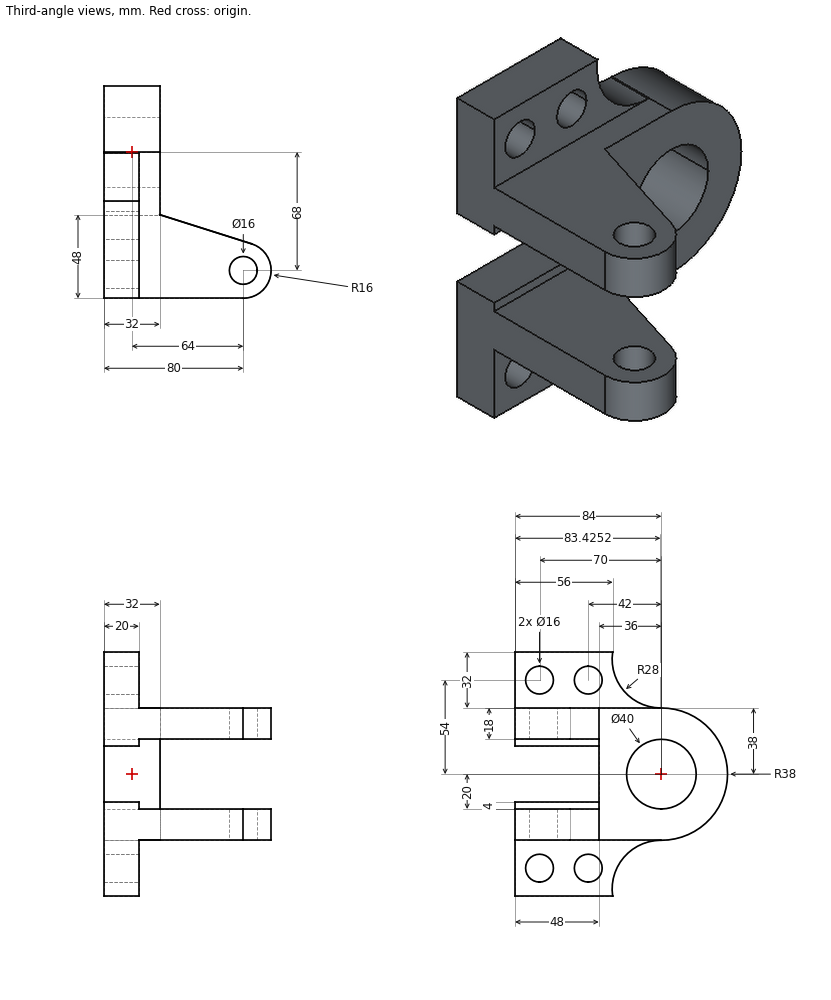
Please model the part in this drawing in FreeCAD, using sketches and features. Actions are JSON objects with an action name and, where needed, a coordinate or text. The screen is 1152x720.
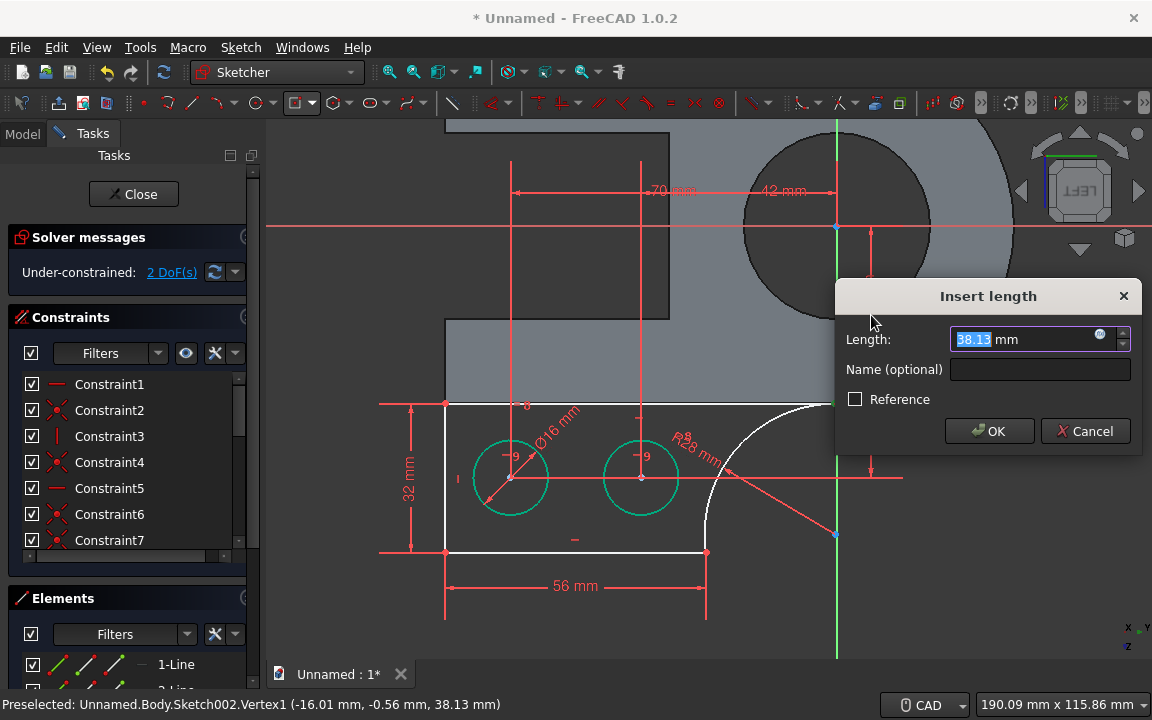
{"action": "type", "text": "38"}
{"action": "key", "text": "Return"}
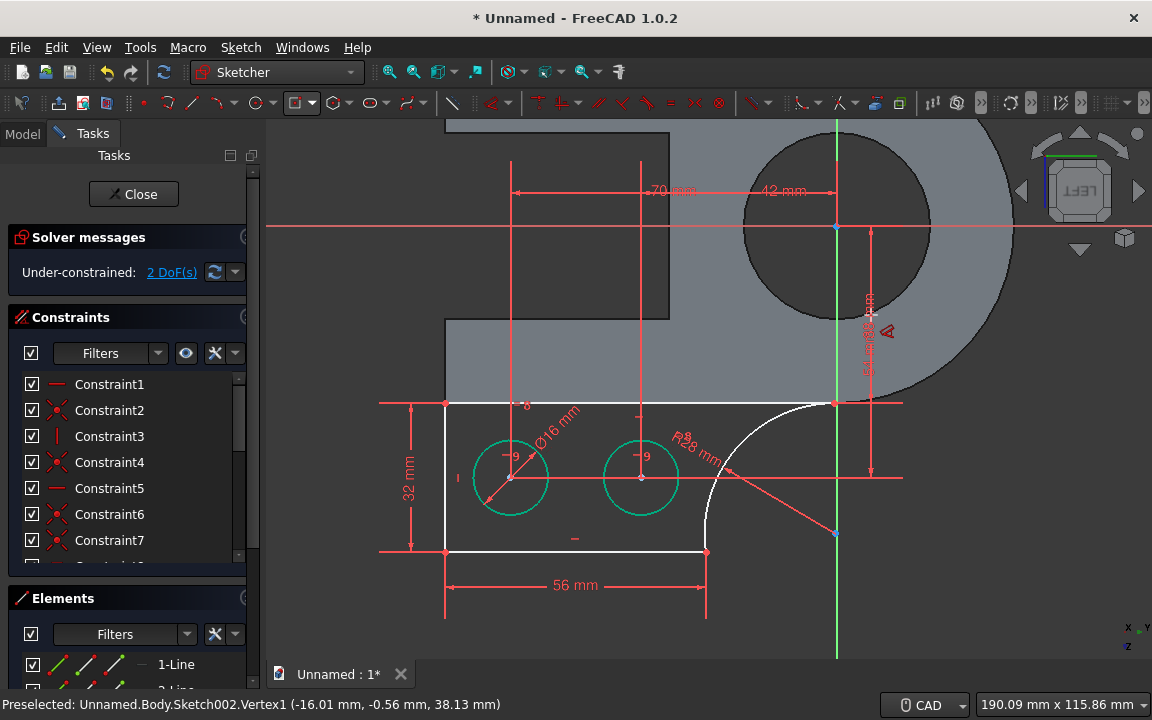
{"action": "left_click", "coordinate": [445, 403]}
{"action": "left_click", "coordinate": [551, 192]}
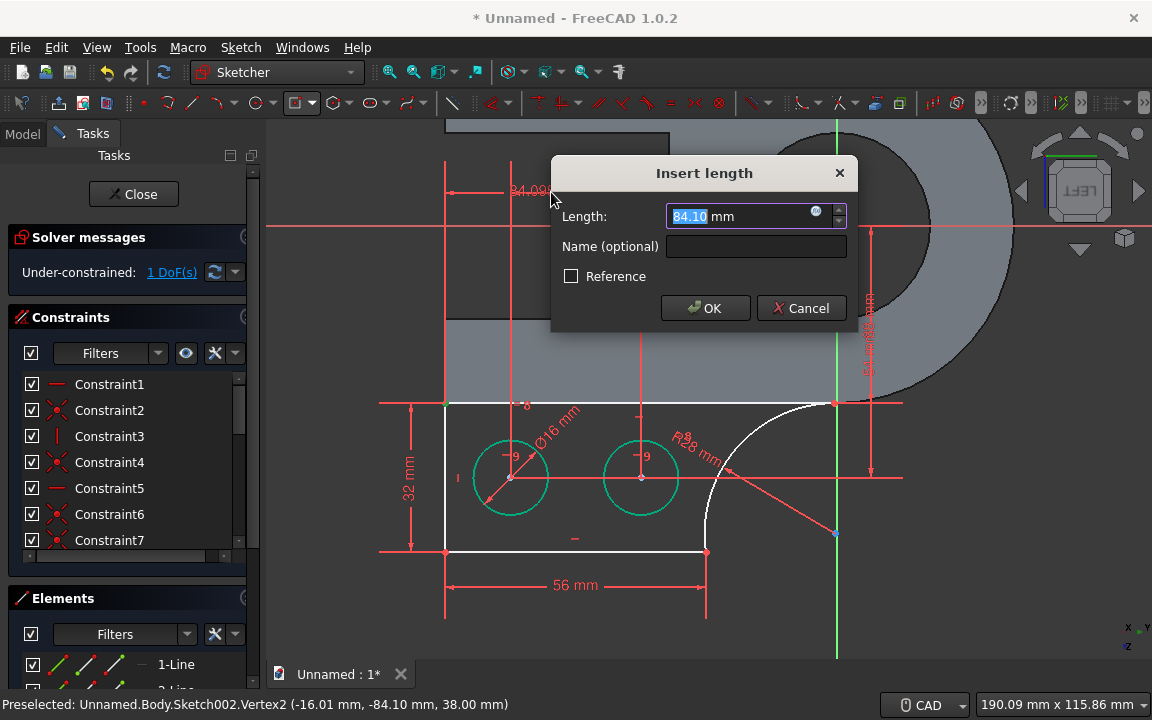
{"action": "type", "text": "84"}
{"action": "key", "text": "Return"}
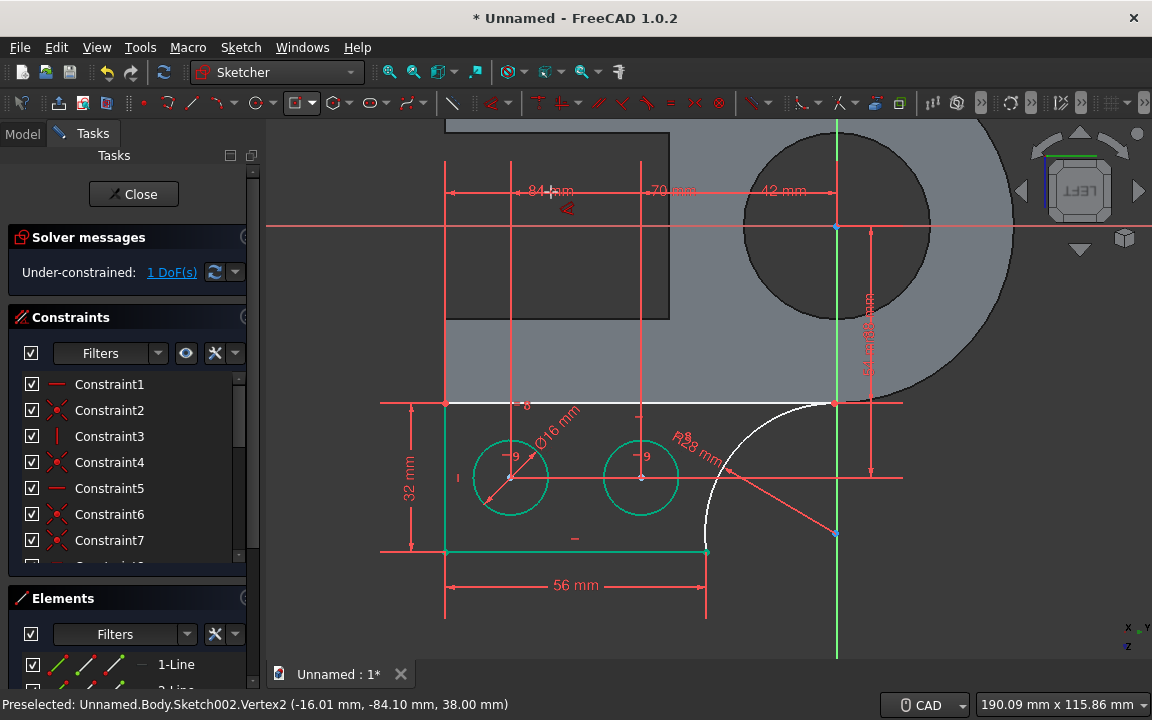
{"action": "left_click", "coordinate": [718, 403]}
{"action": "left_click", "coordinate": [776, 437]}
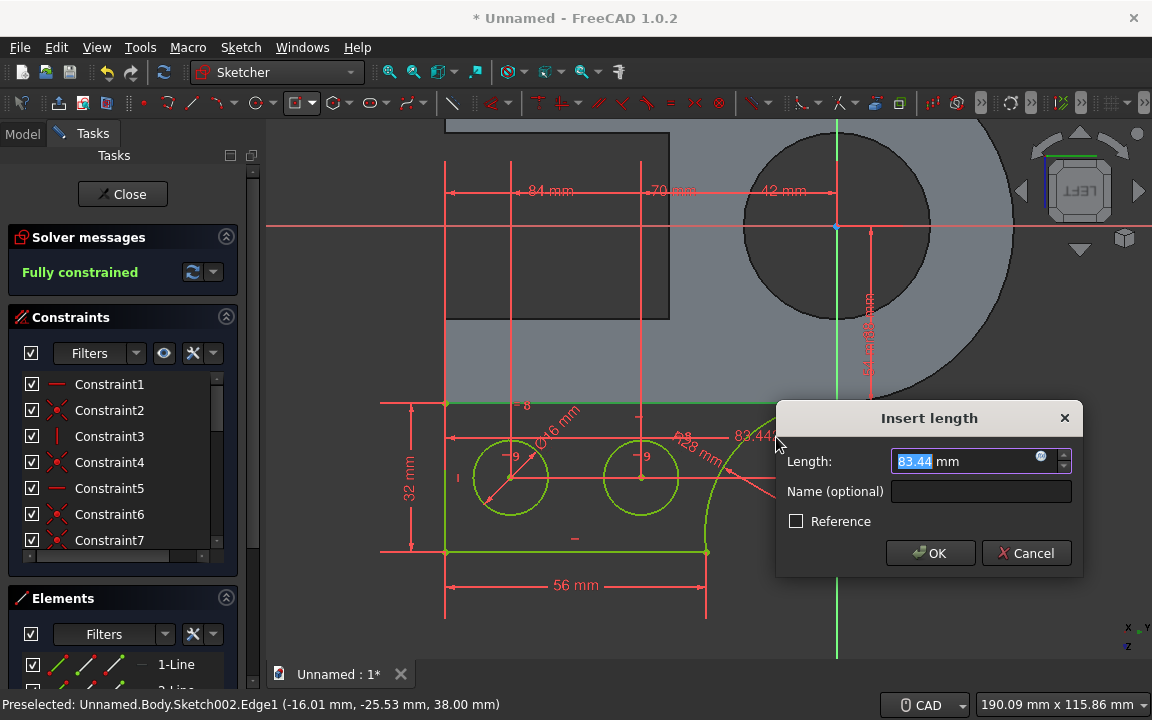
{"action": "type", "text": "83.4252"}
{"action": "key", "text": "Return"}
{"action": "key", "text": "Escape"}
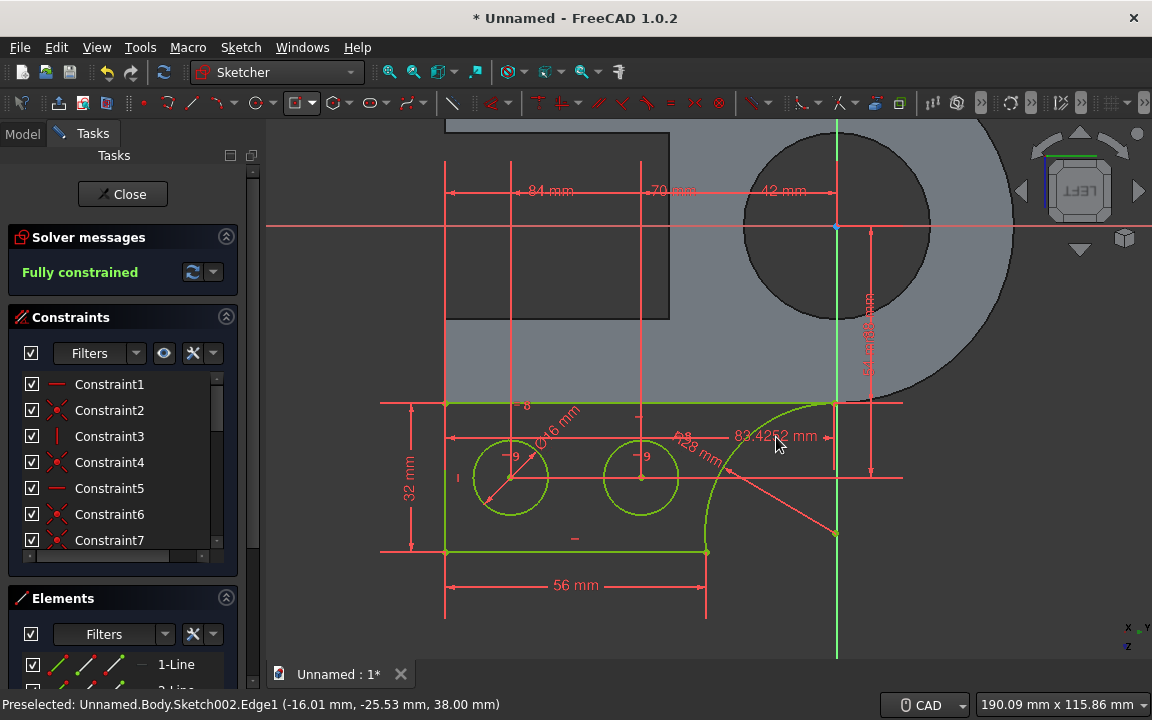
{"action": "left_click", "coordinate": [123, 194]}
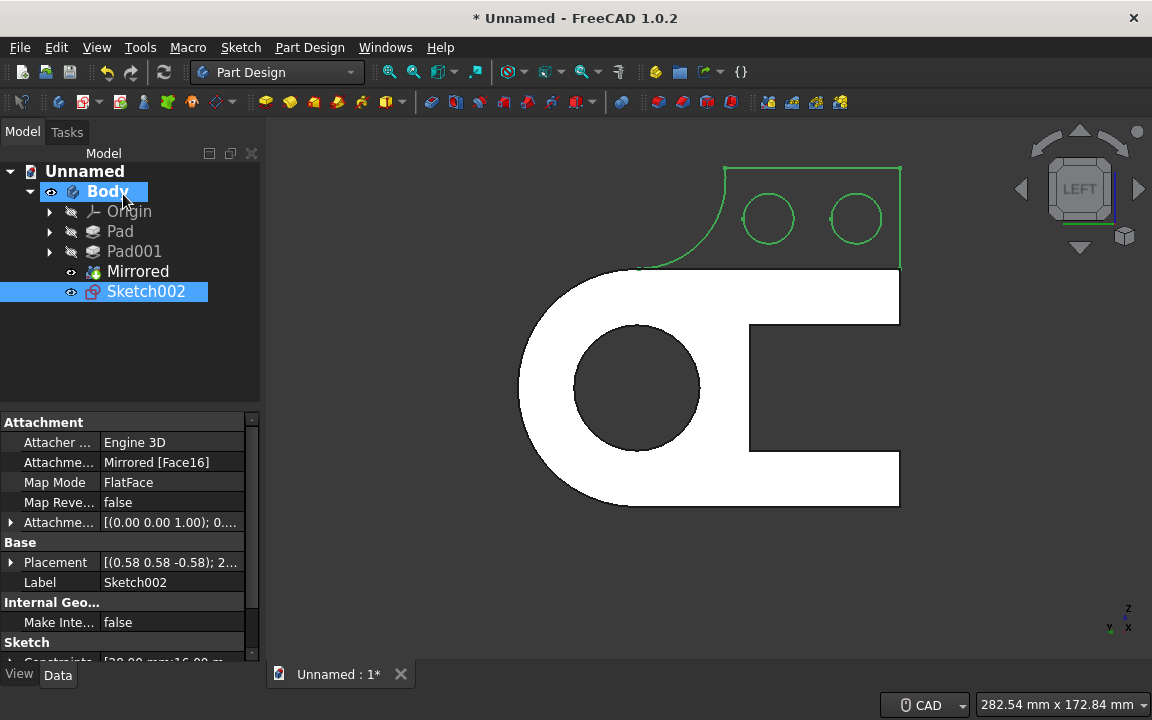
{"action": "left_click", "coordinate": [266, 102]}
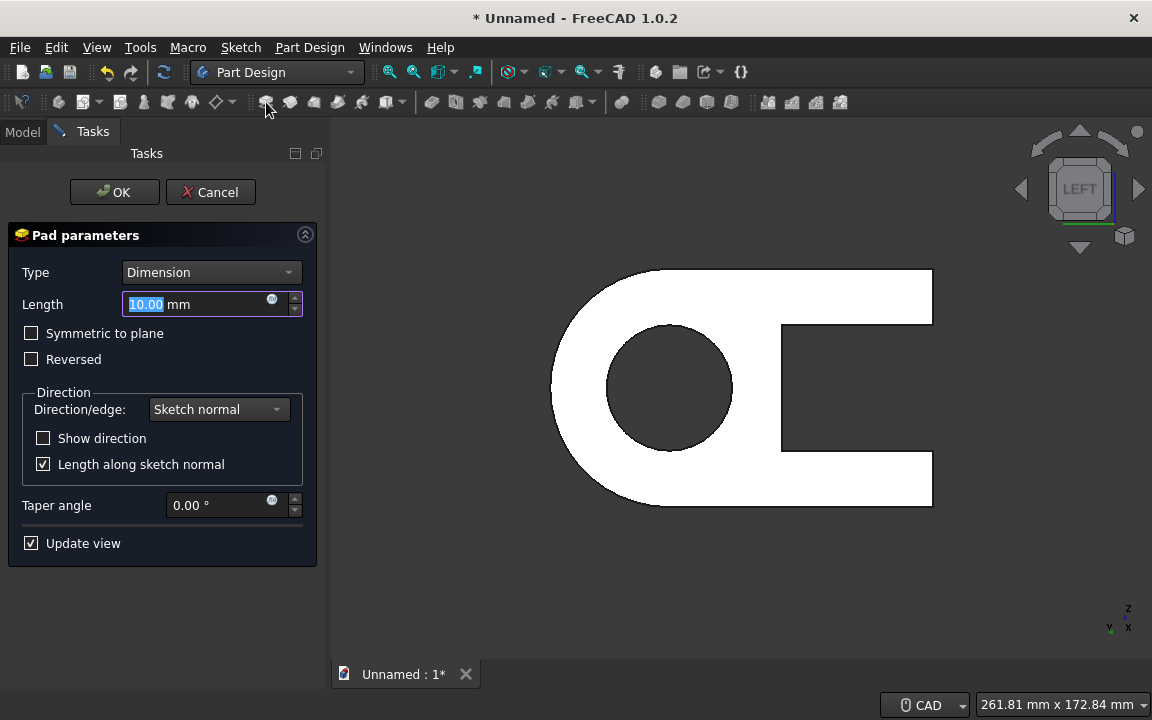
{"action": "type", "text": "20"}
{"action": "key", "text": "Tab"}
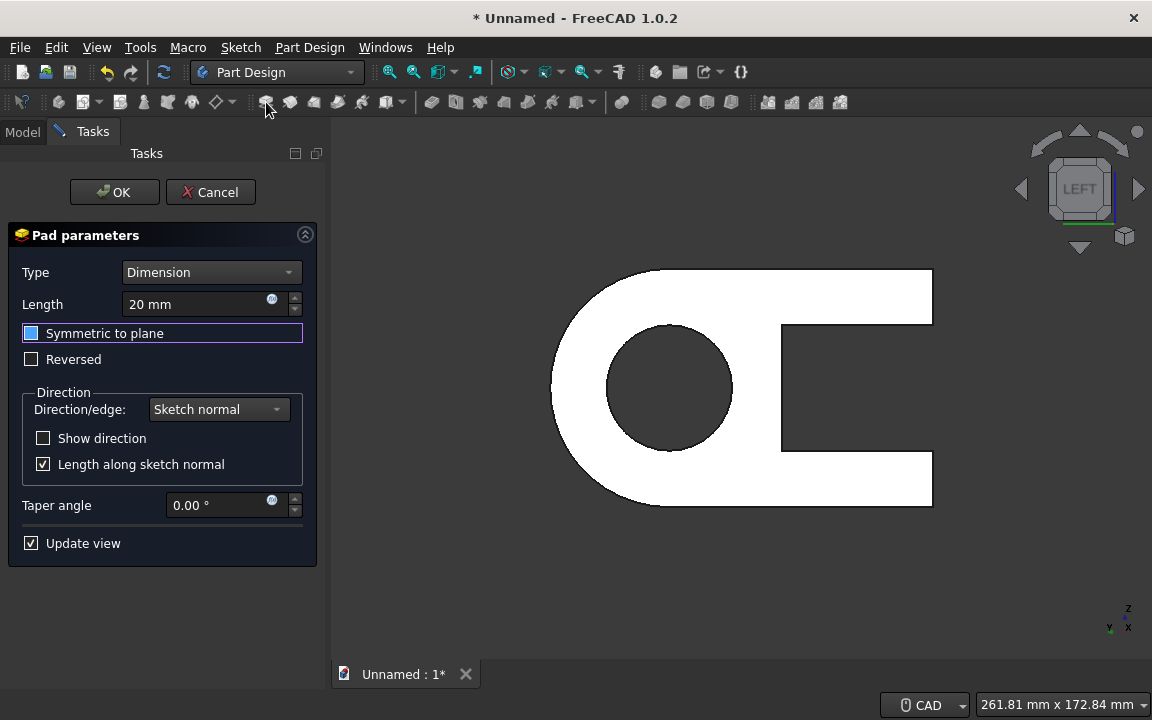
{"action": "left_click", "coordinate": [30, 359]}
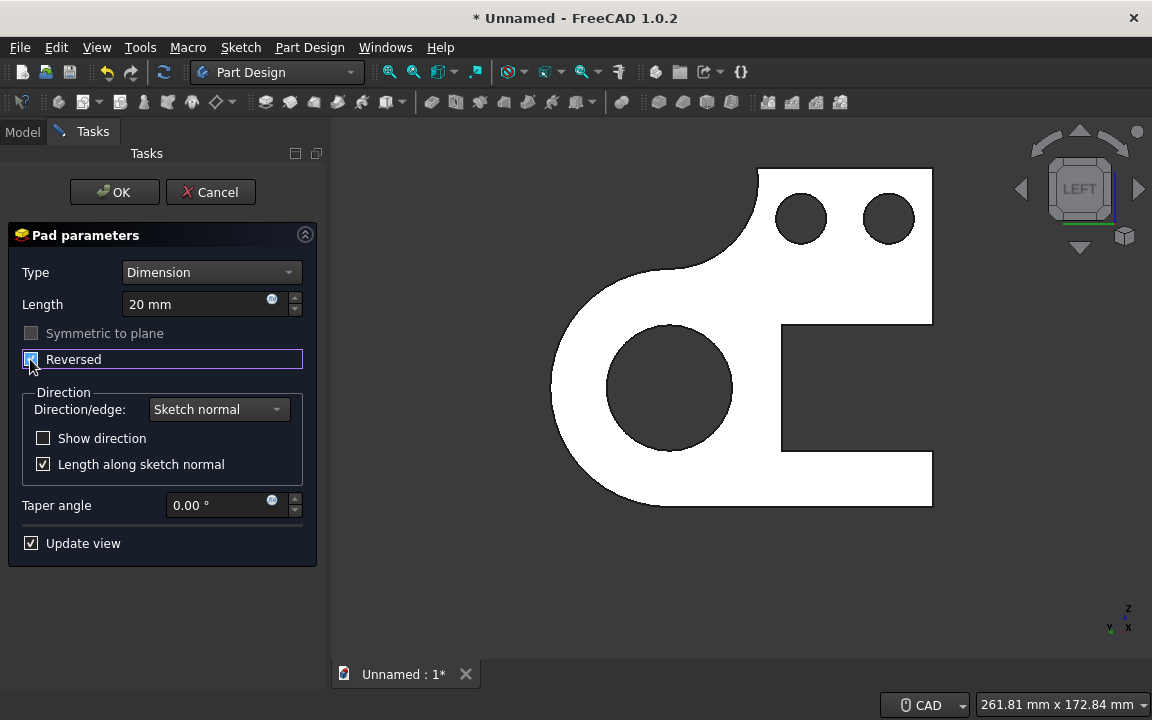
{"action": "left_click", "coordinate": [115, 192]}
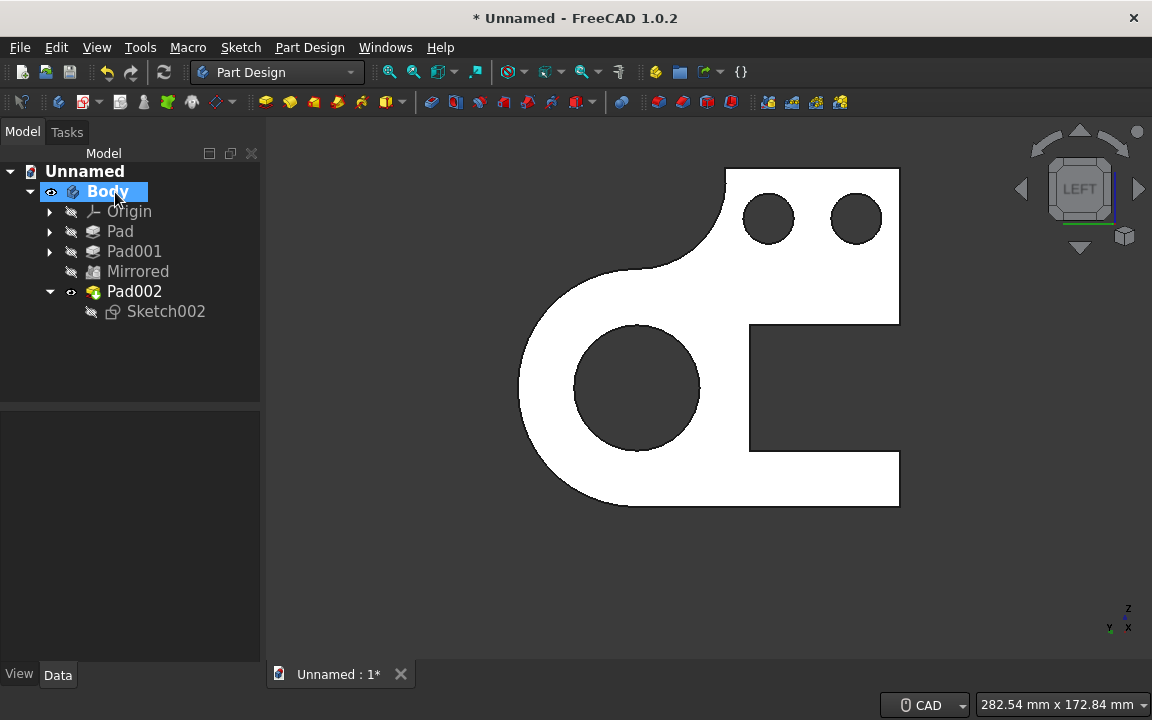
{"action": "left_click", "coordinate": [116, 292]}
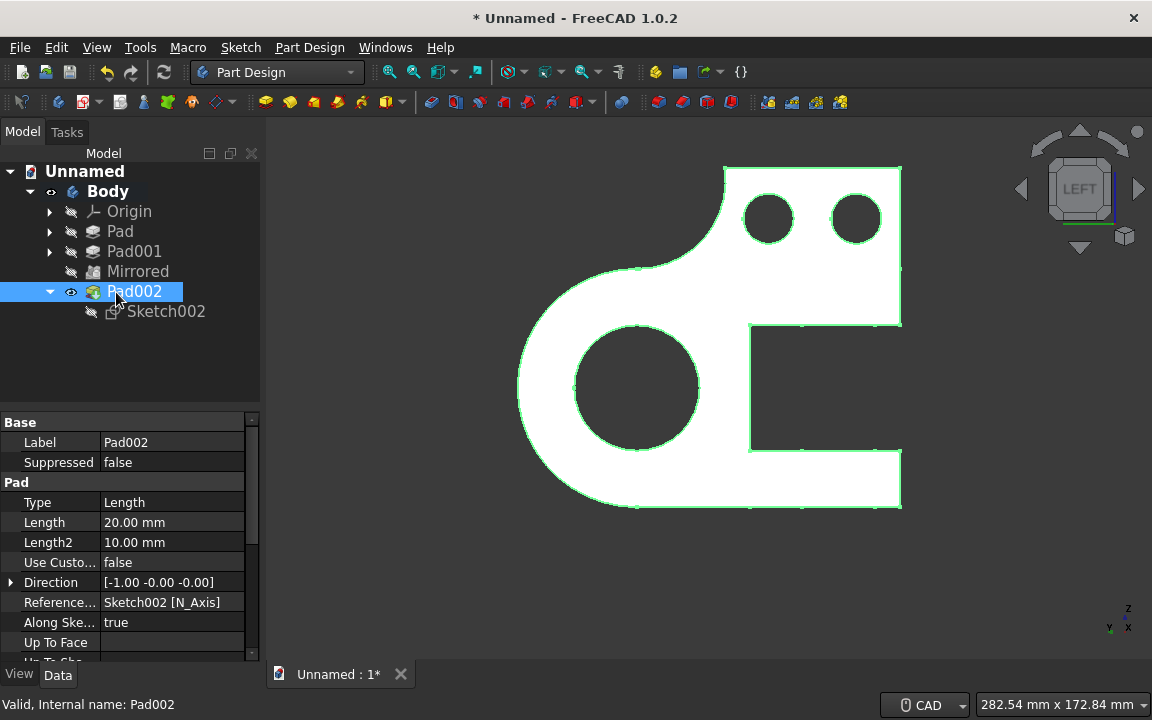
{"action": "left_click", "coordinate": [768, 102]}